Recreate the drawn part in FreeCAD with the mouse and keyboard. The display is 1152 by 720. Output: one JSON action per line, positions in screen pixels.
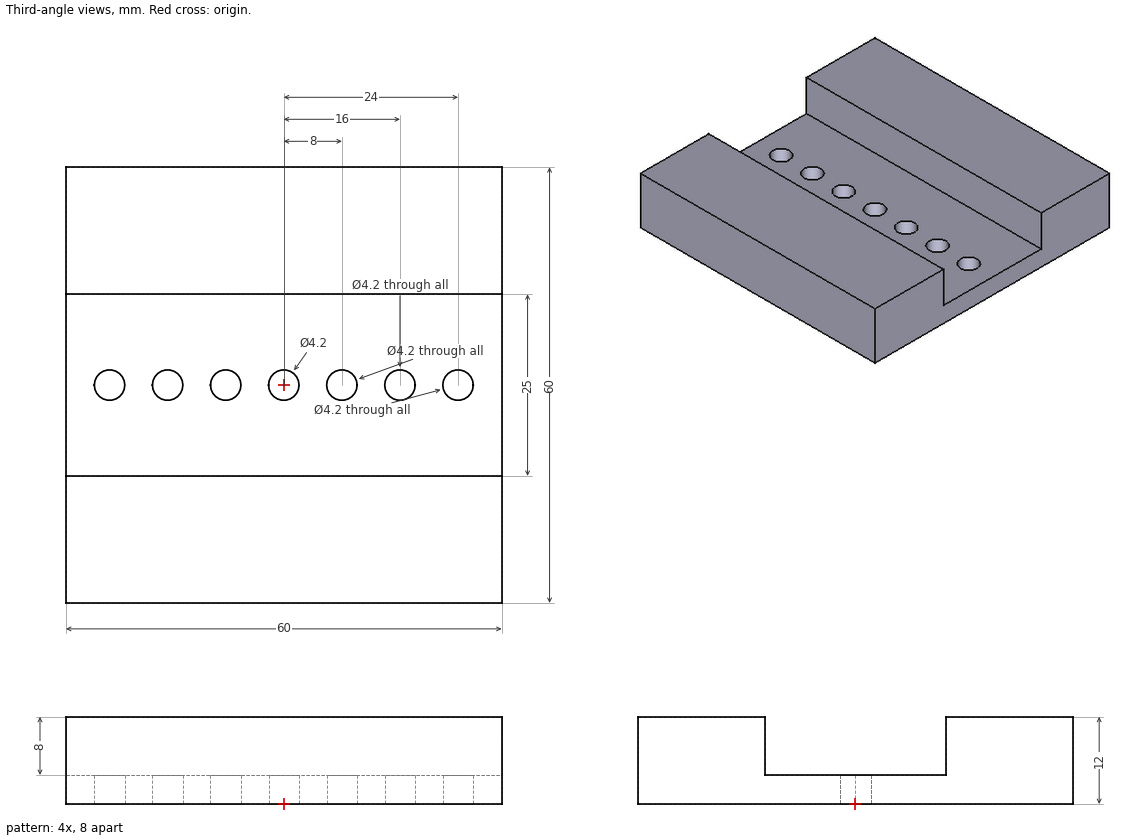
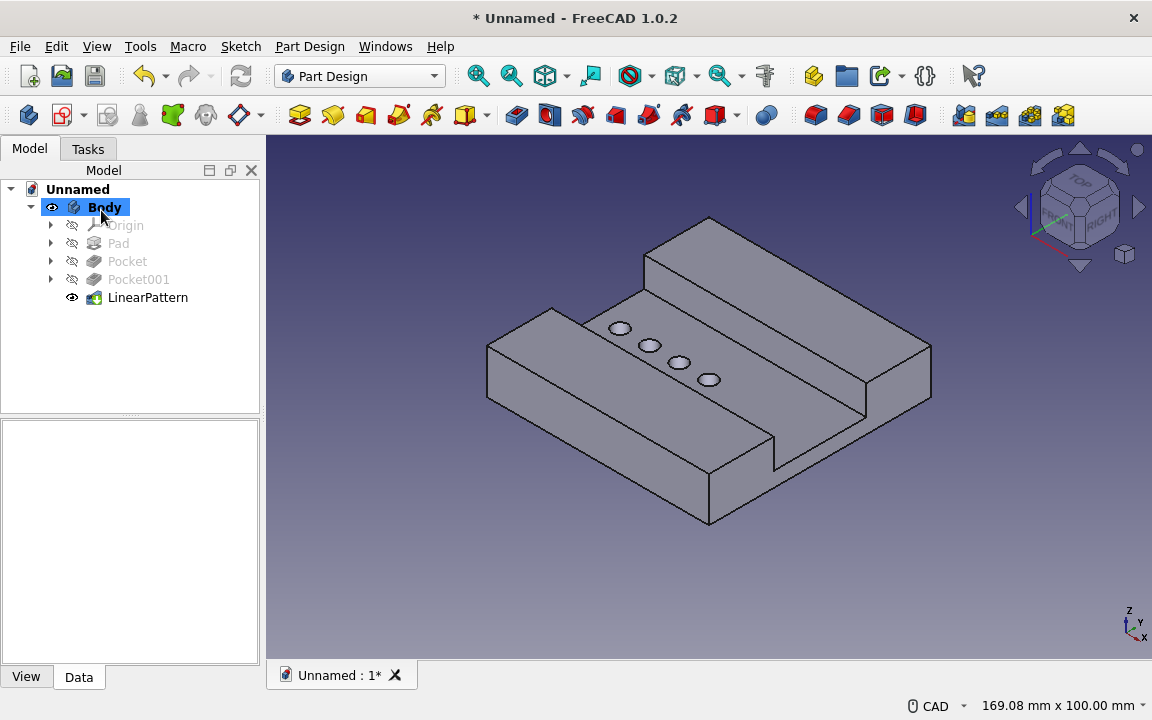
{"action": "left_click", "coordinate": [773, 416]}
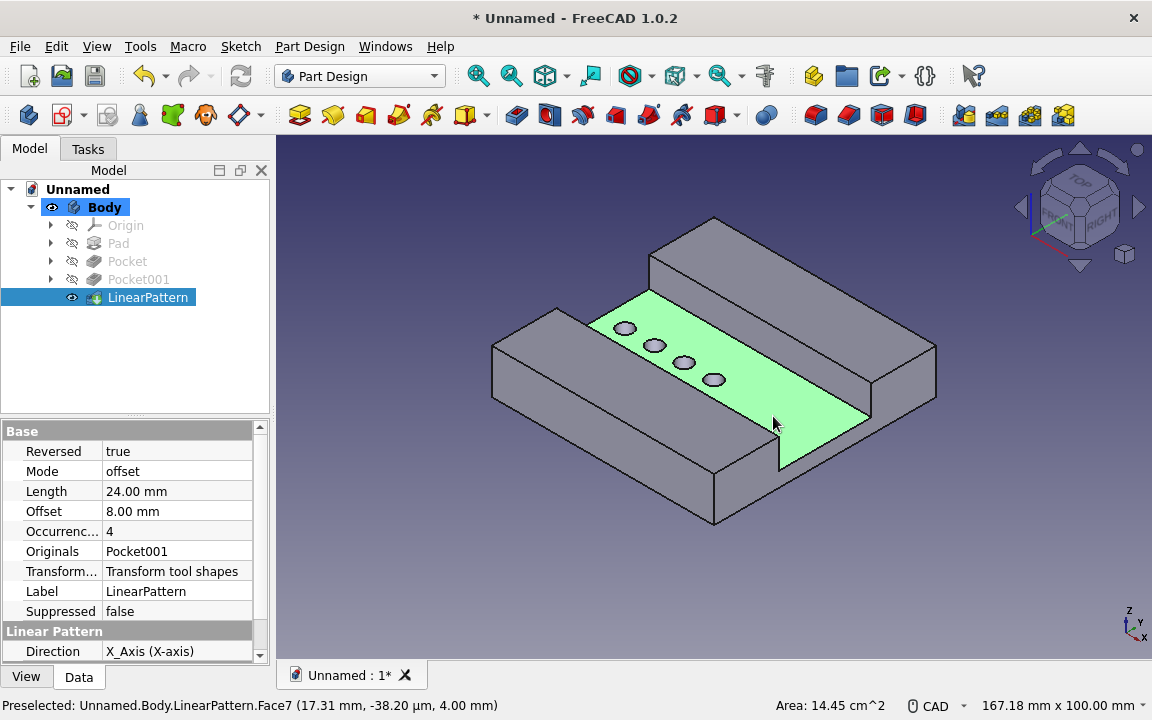
{"action": "left_click", "coordinate": [62, 116]}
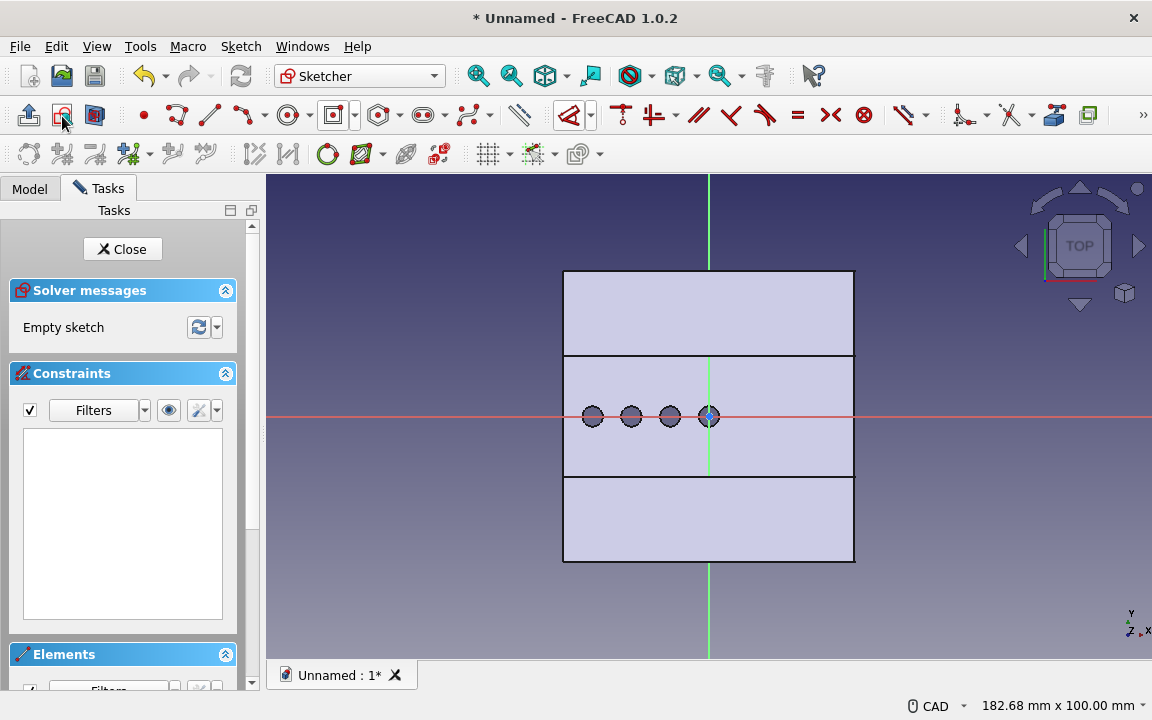
{"action": "left_click", "coordinate": [95, 116]}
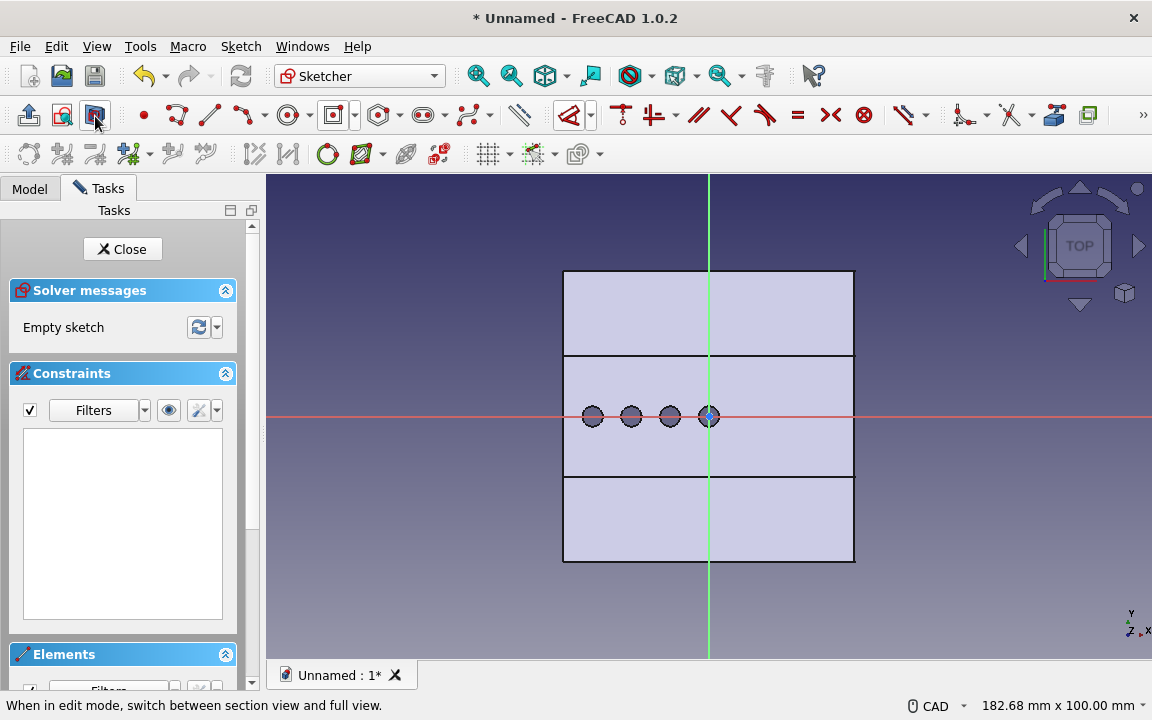
{"action": "scroll", "coordinate": [743, 416], "scroll_direction": "up", "scroll_amount": 12}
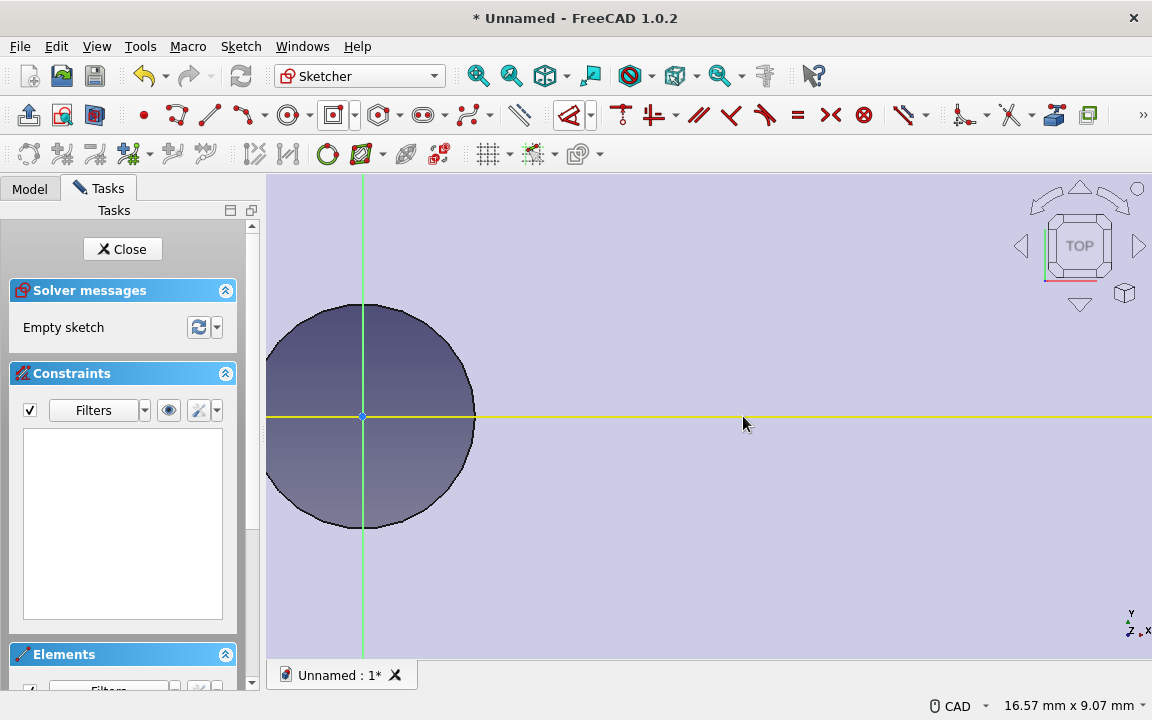
{"action": "left_click", "coordinate": [288, 116]}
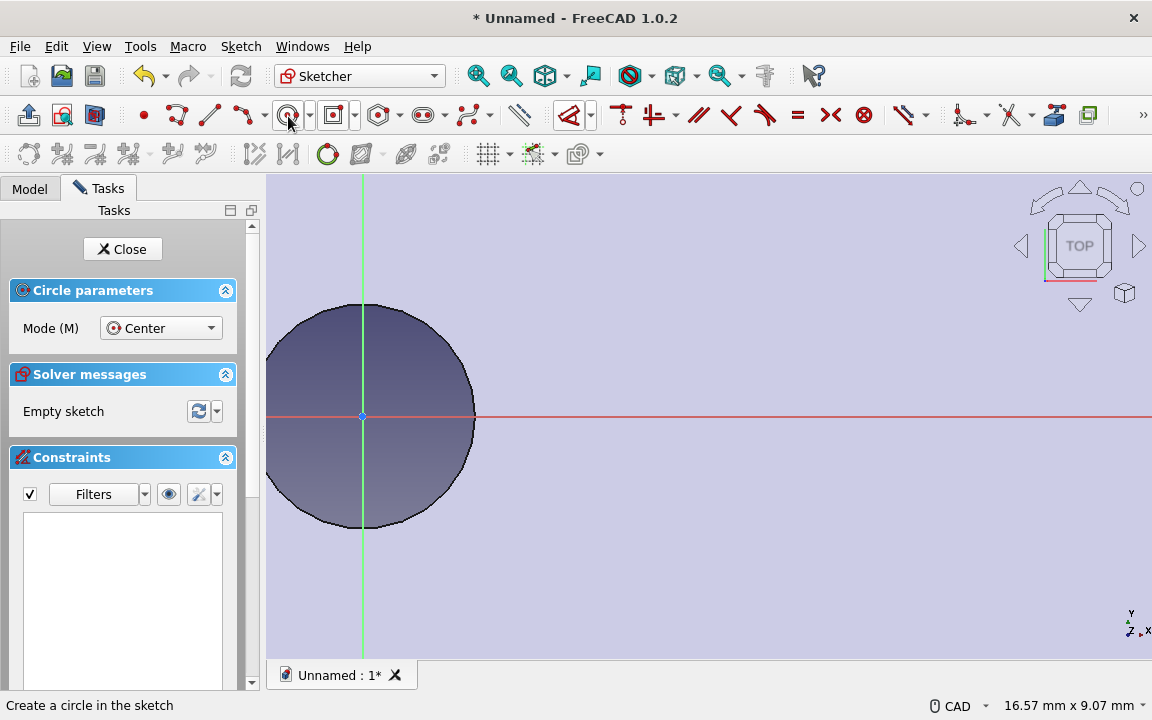
{"action": "left_click", "coordinate": [791, 416]}
{"action": "mouse_move", "coordinate": [870, 337]}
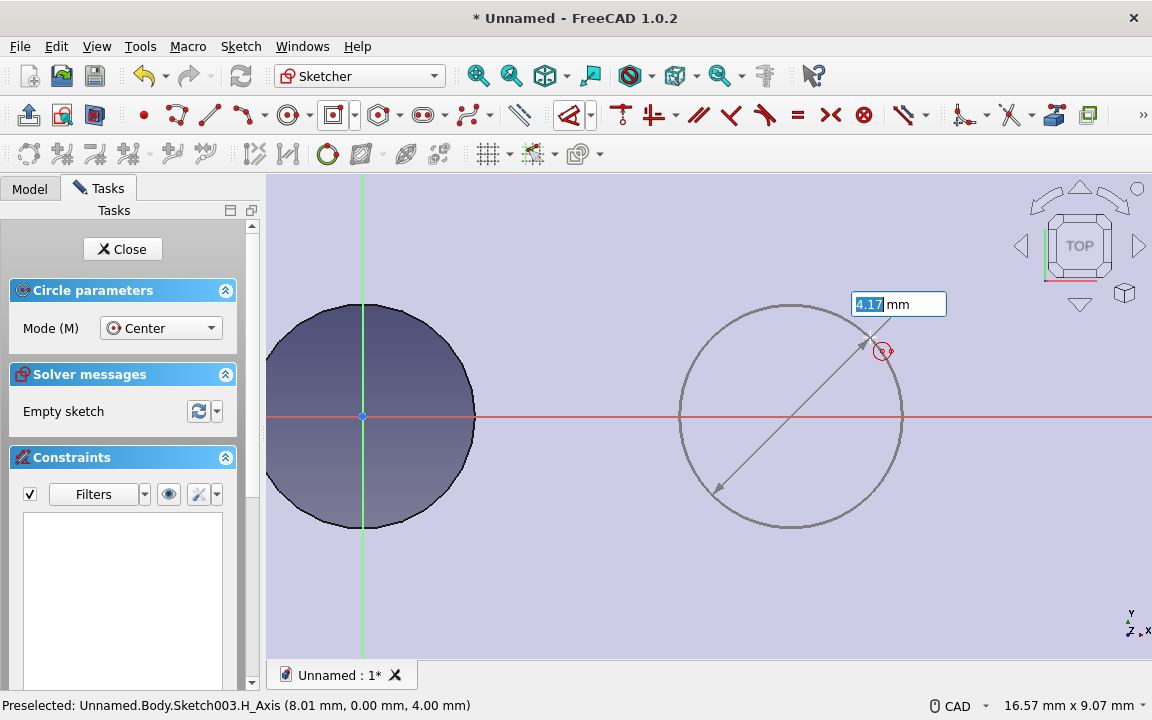
{"action": "type", "text": "4.2"}
{"action": "key", "text": "Return"}
{"action": "key", "text": "Escape"}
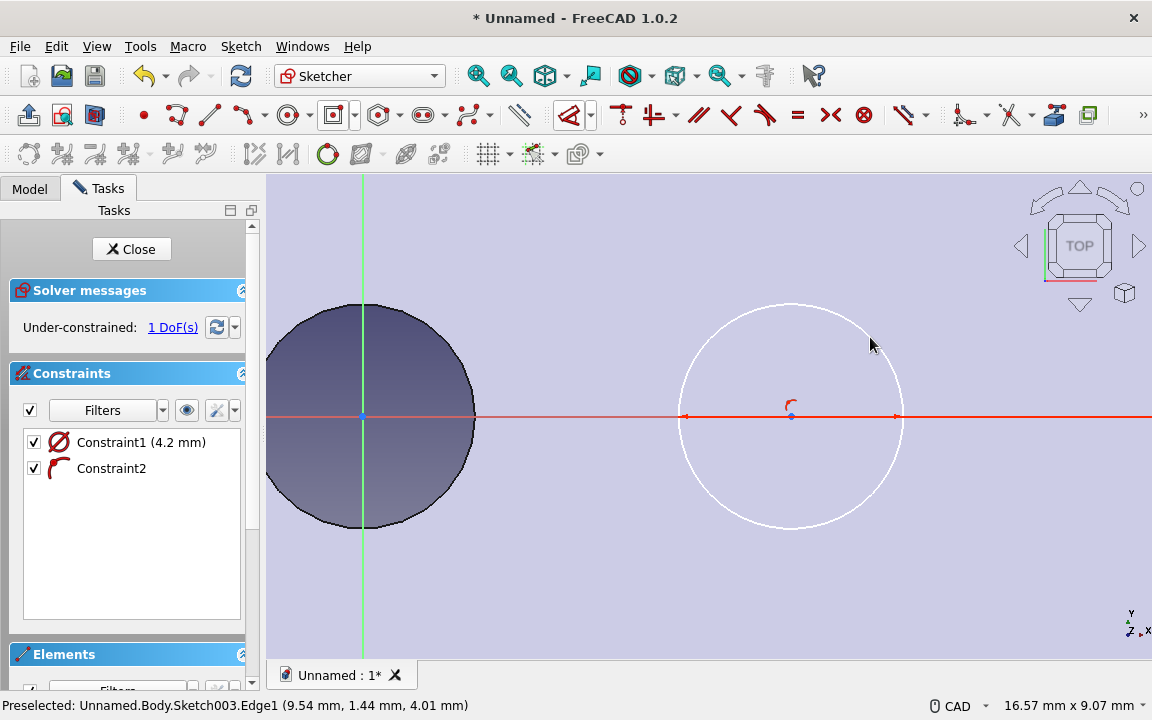
{"action": "left_click", "coordinate": [791, 416]}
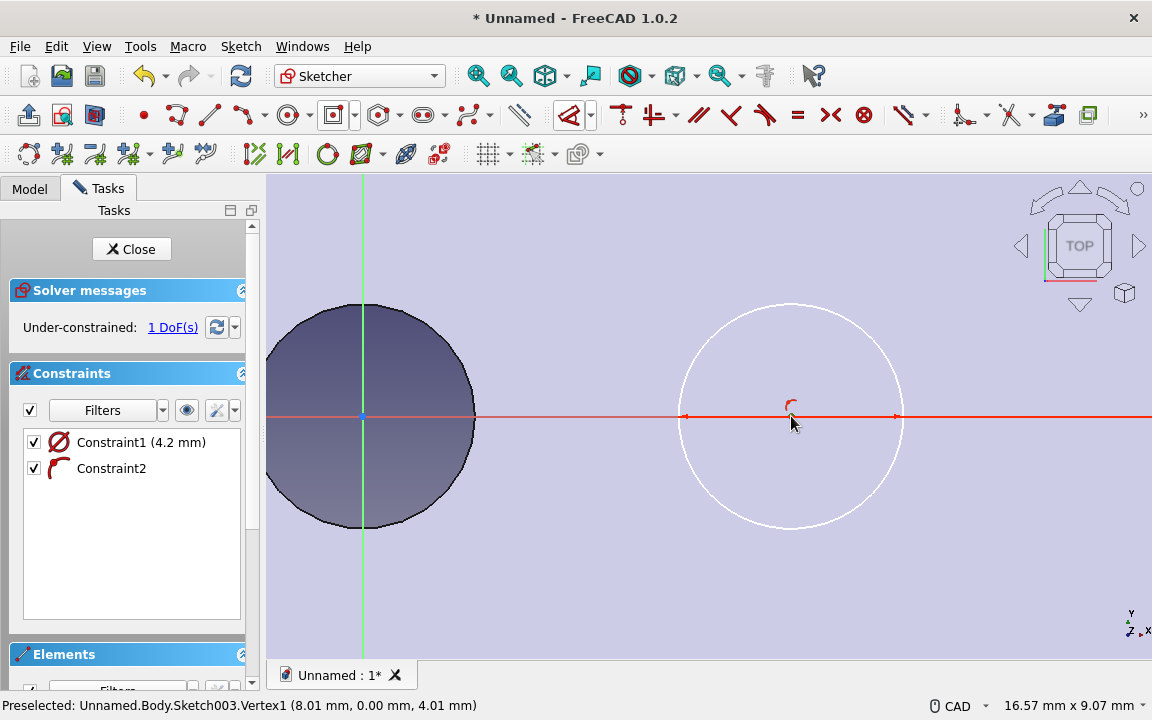
{"action": "left_click", "coordinate": [590, 116]}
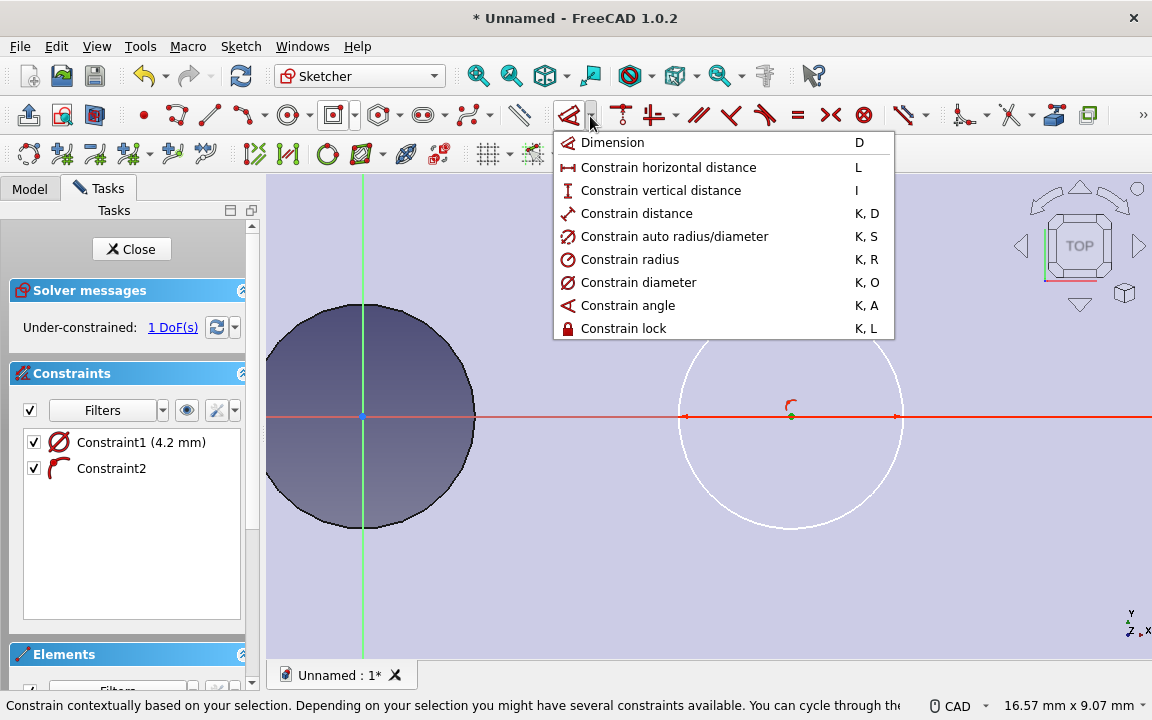
{"action": "left_click", "coordinate": [724, 168]}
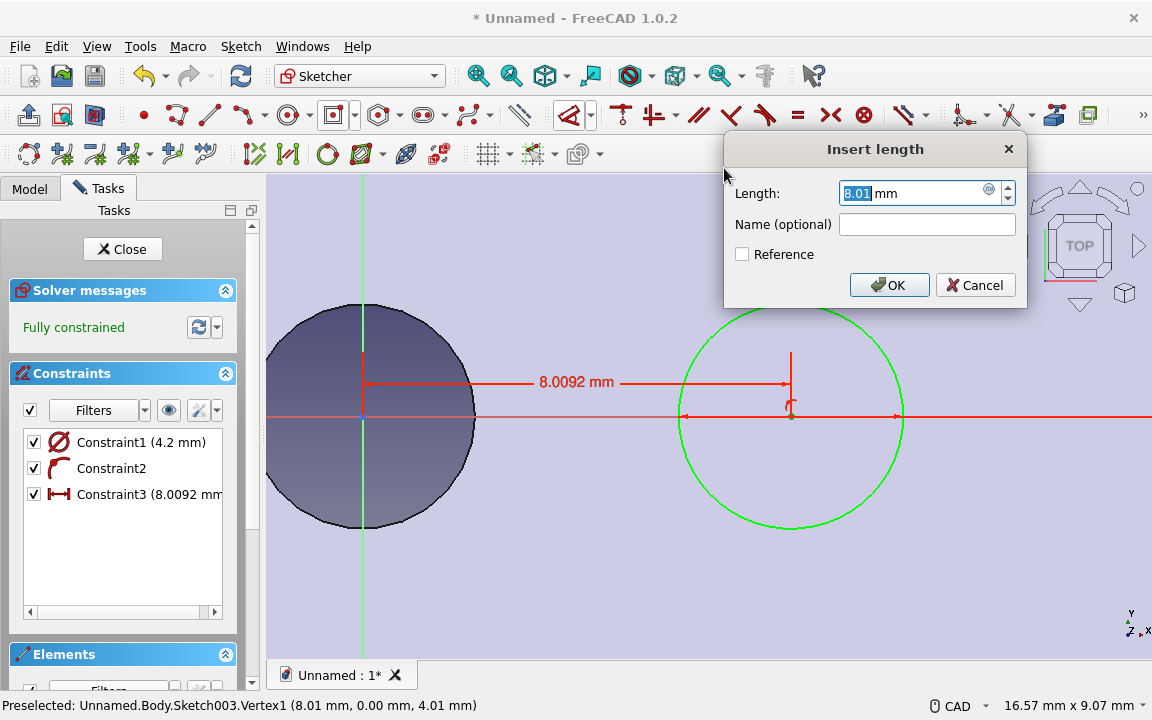
{"action": "type", "text": "8"}
{"action": "key", "text": "Return"}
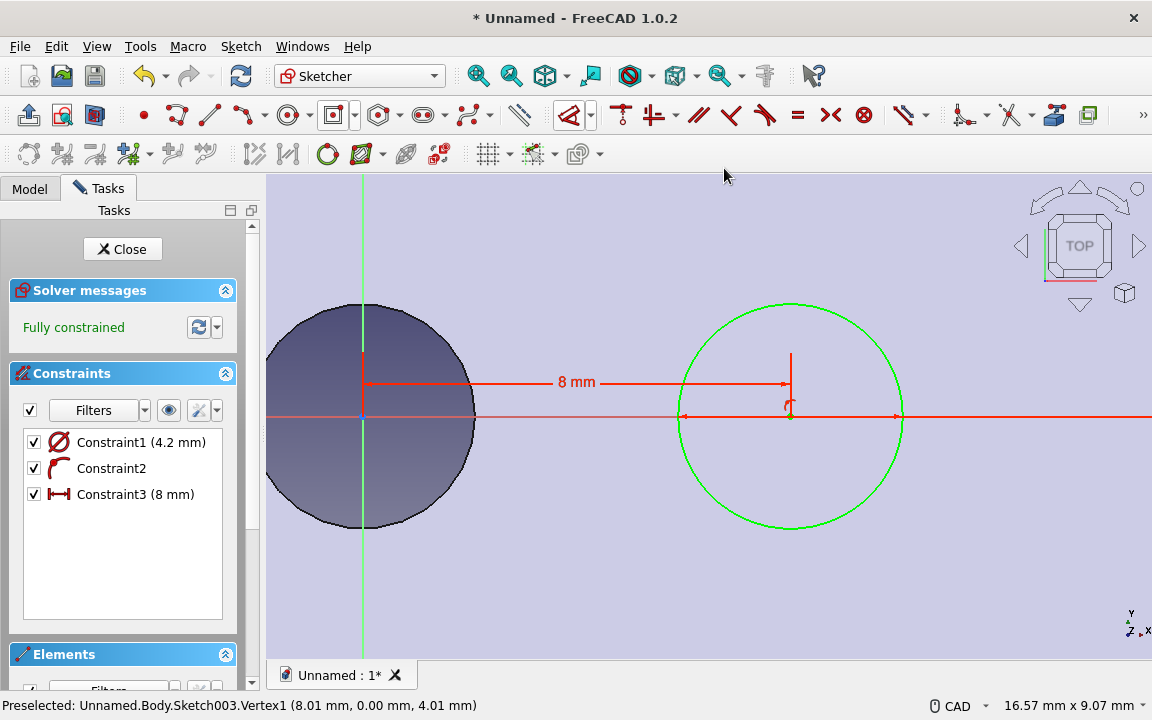
{"action": "left_click", "coordinate": [123, 249]}